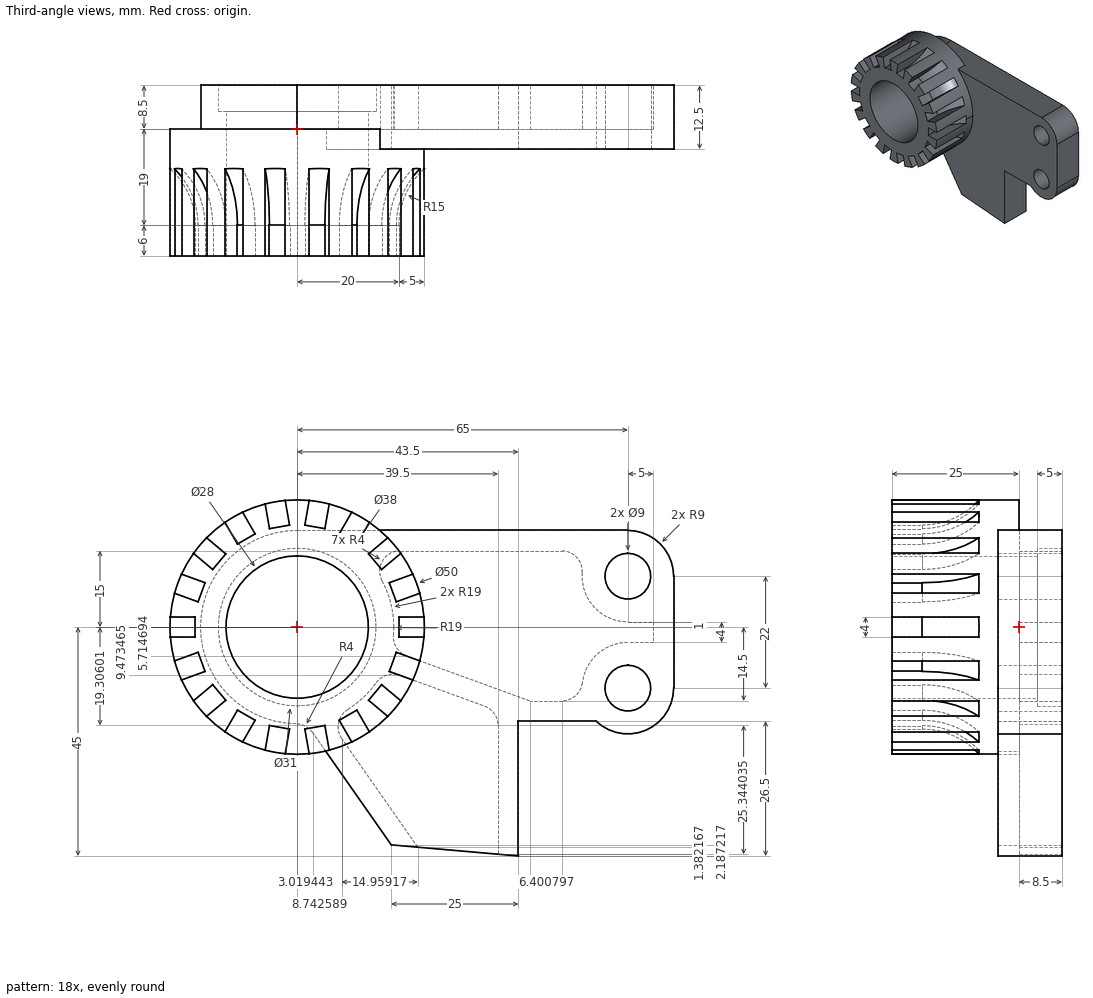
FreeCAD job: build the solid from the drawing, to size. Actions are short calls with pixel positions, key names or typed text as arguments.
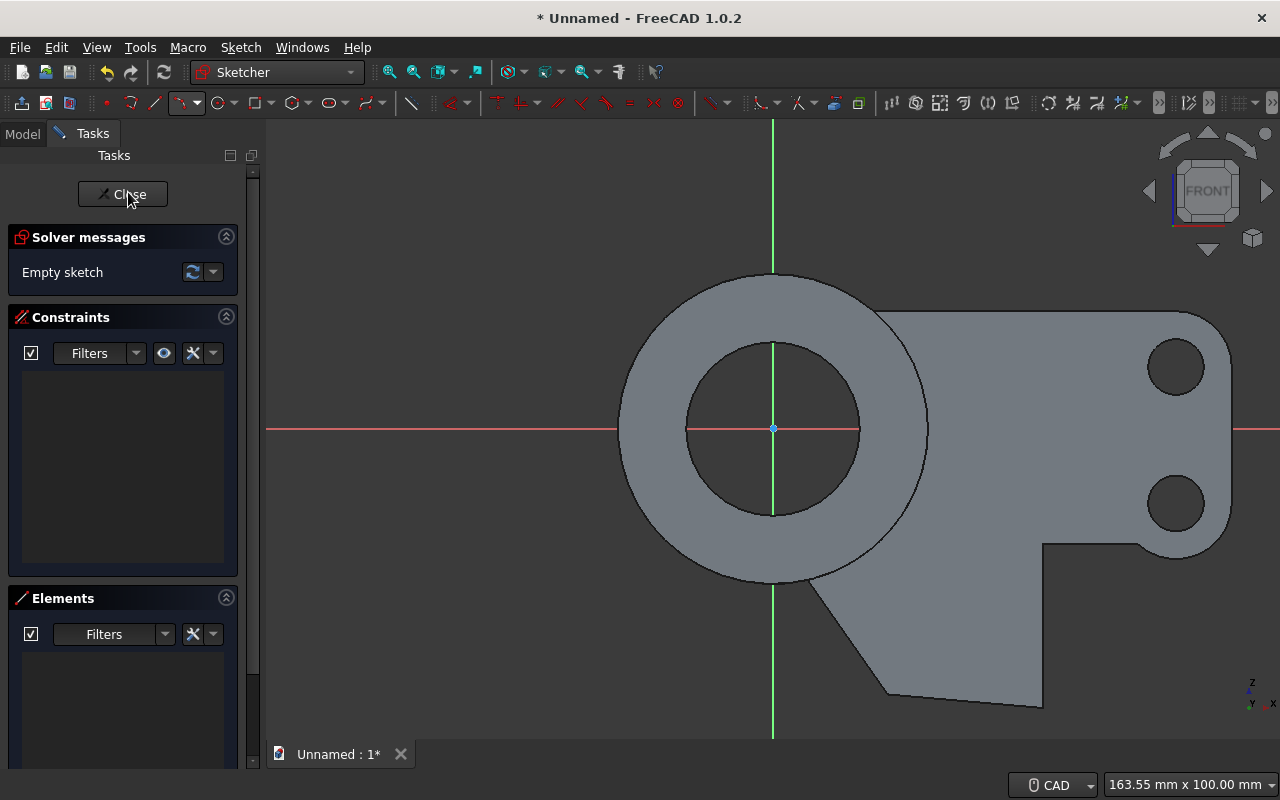
click(70, 104)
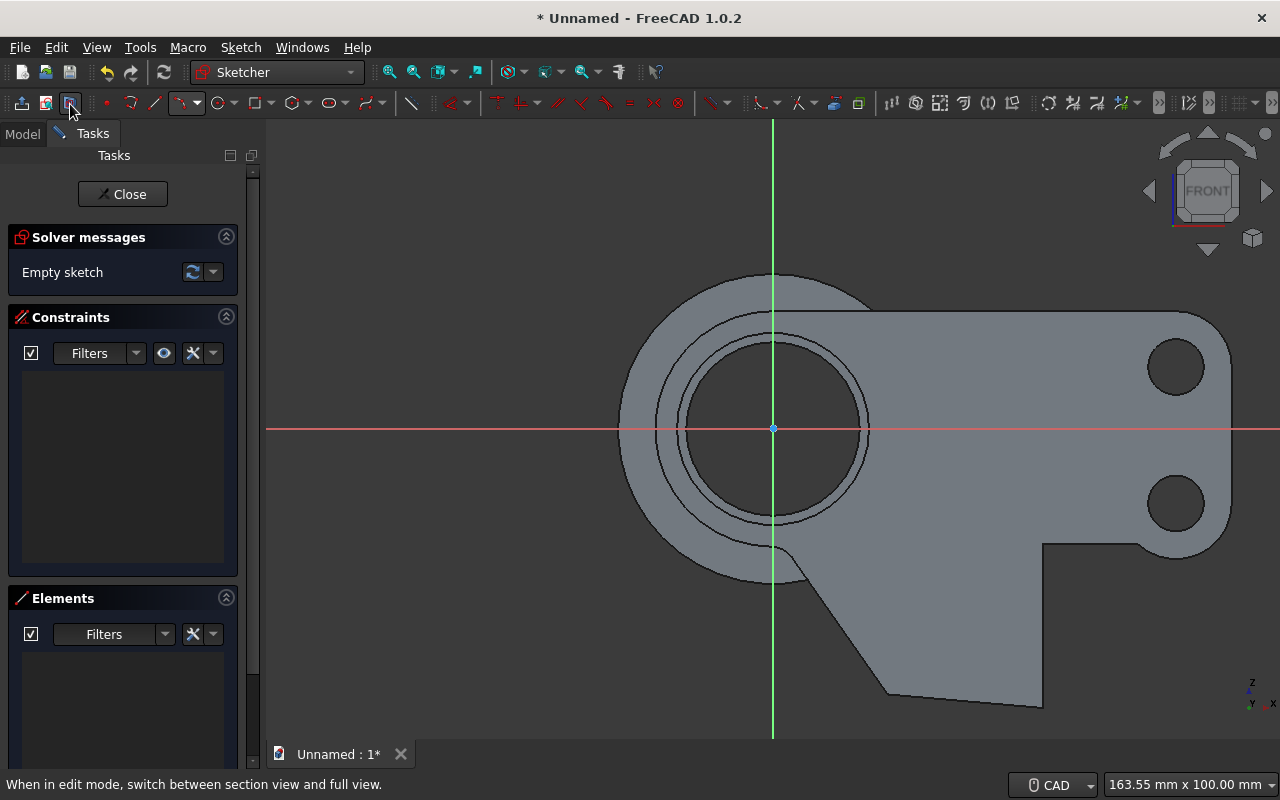
scroll(294, 147, down, 1)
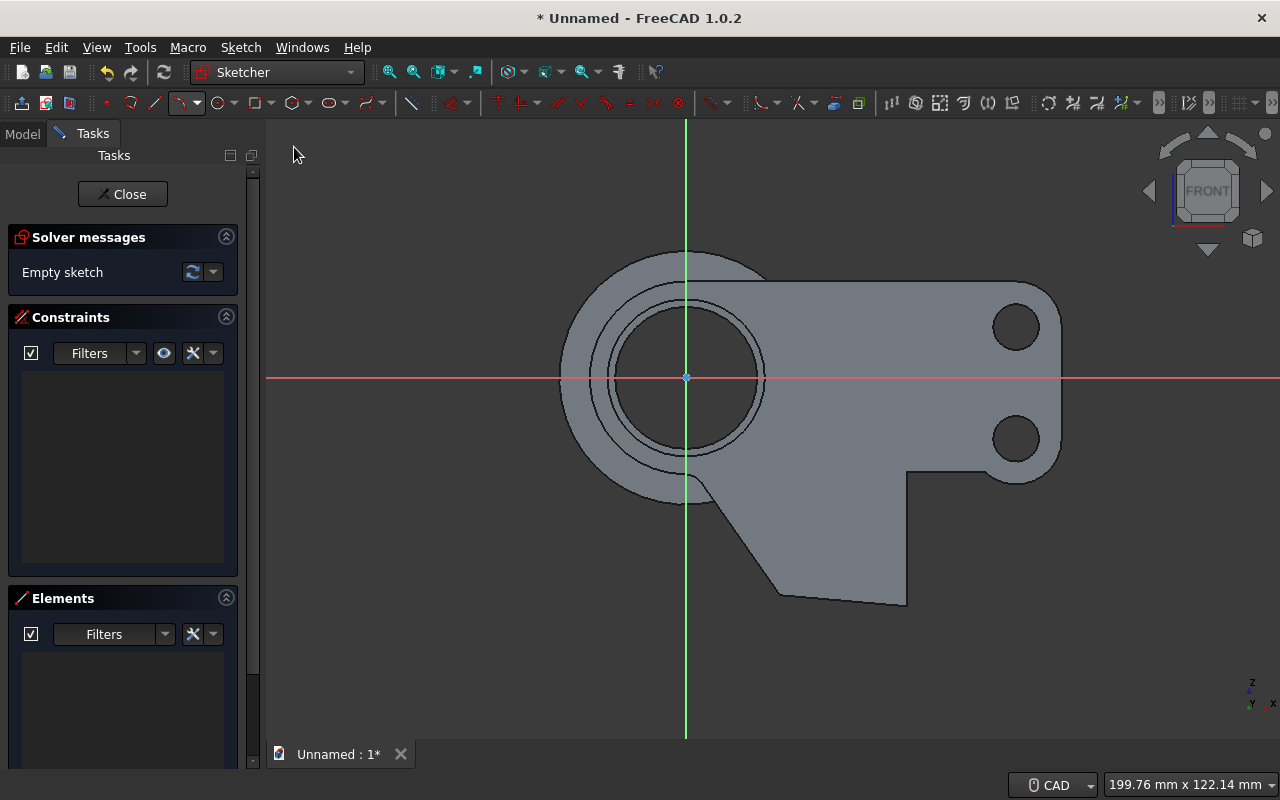
click(156, 104)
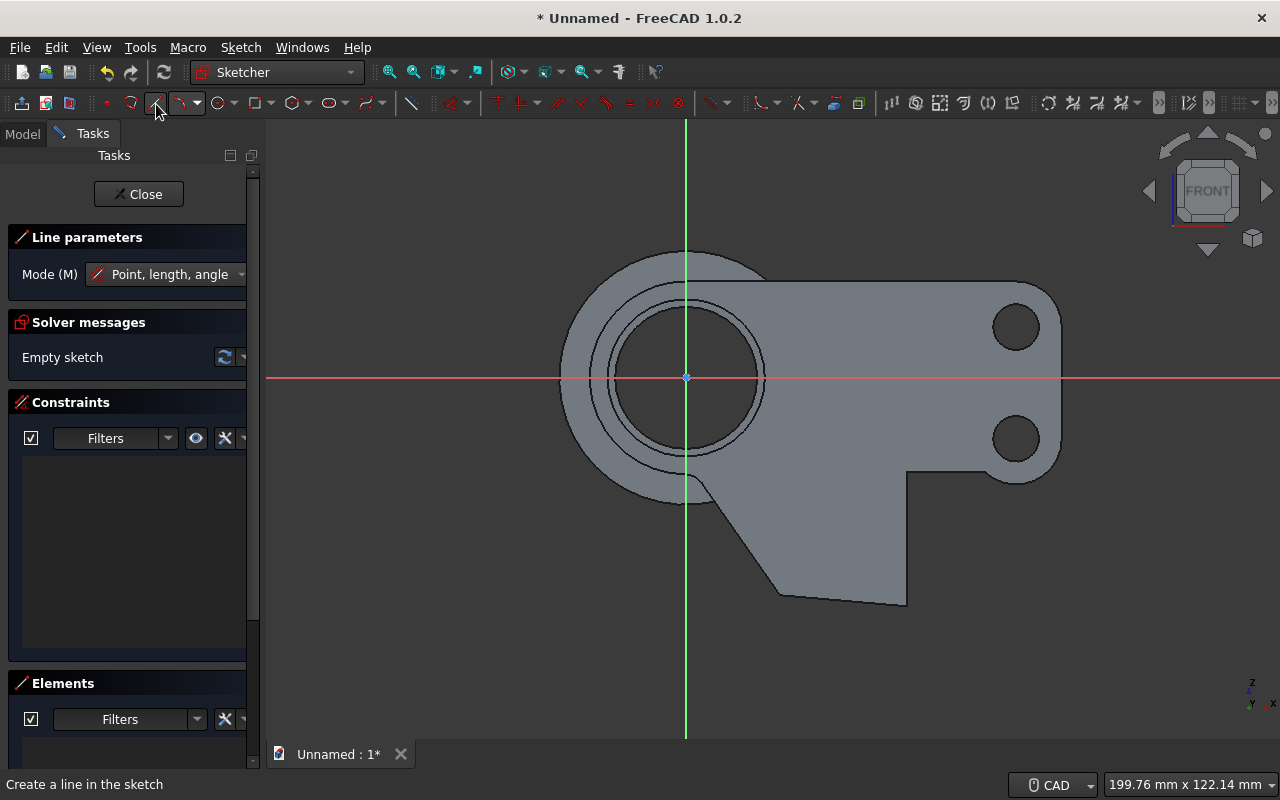
click(789, 302)
click(950, 302)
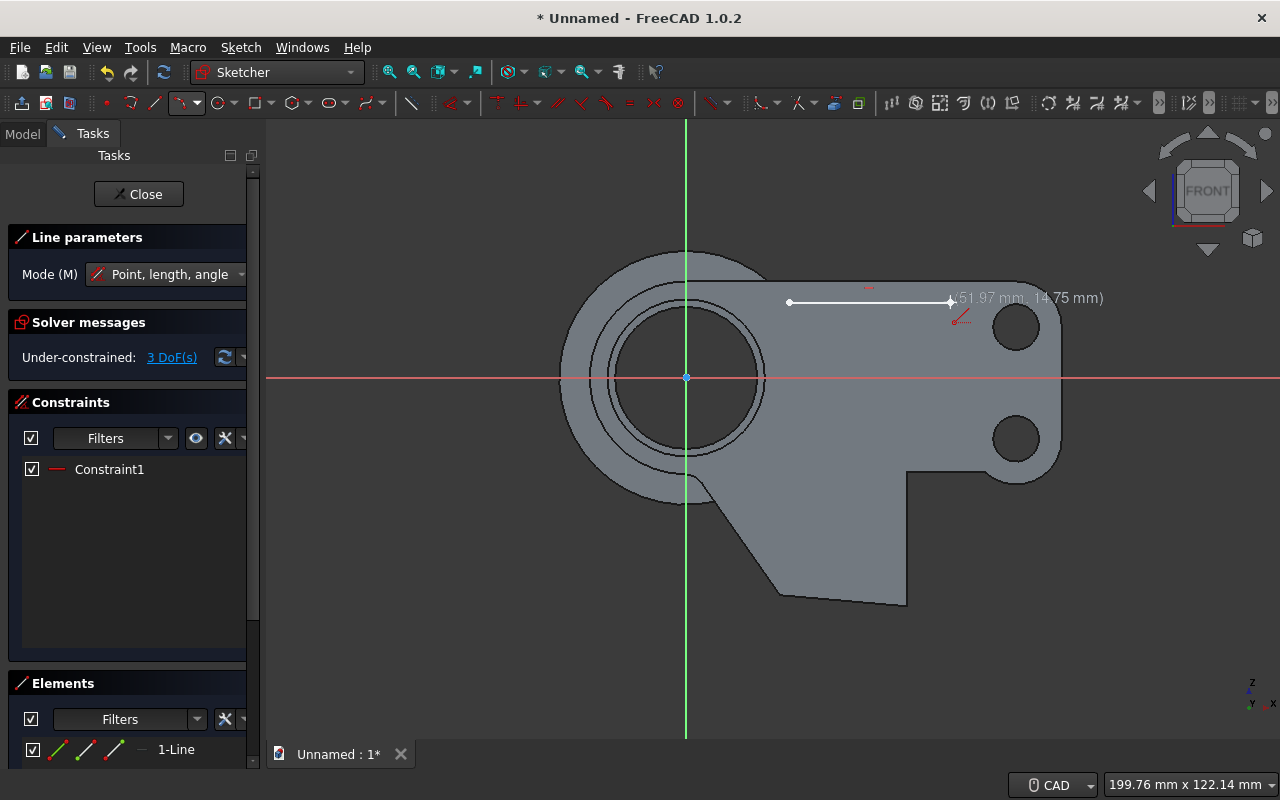
click(132, 104)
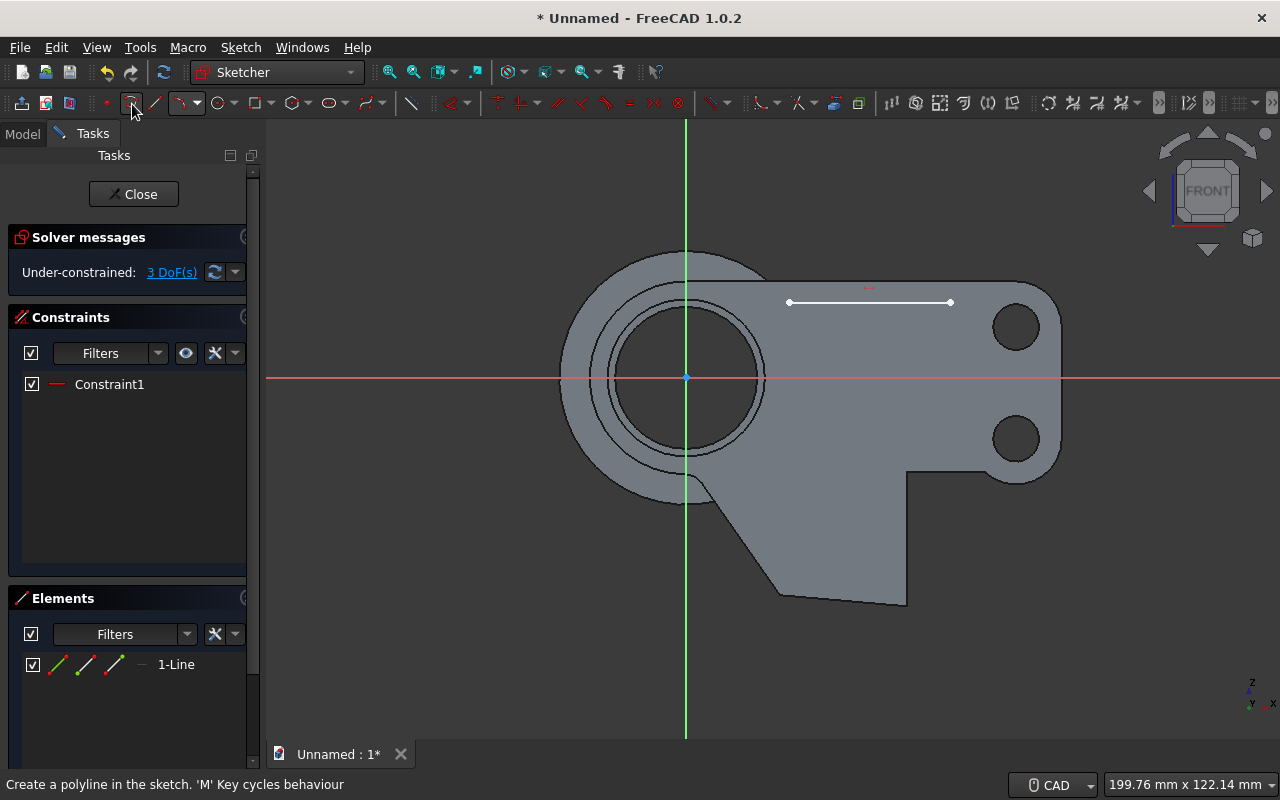
scroll(1016, 373, up, 6)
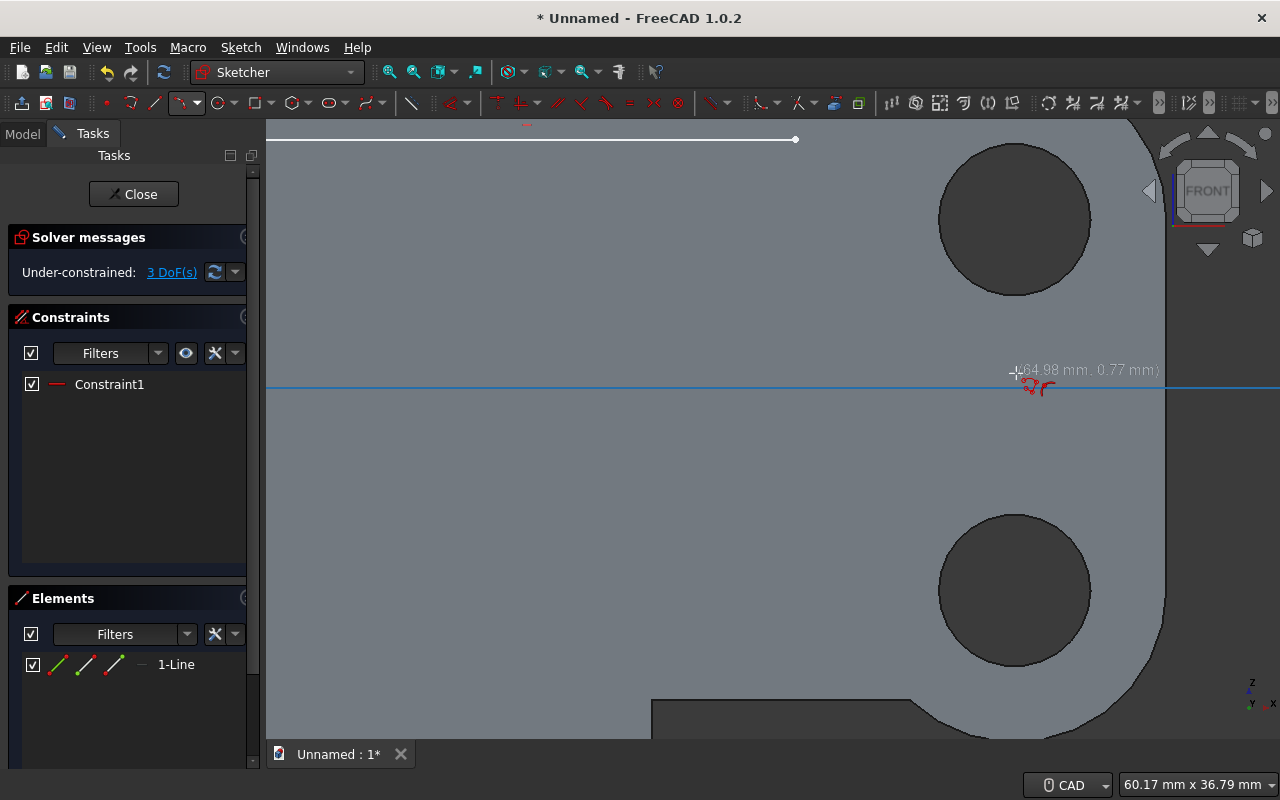
click(1015, 371)
click(1099, 371)
click(1099, 439)
click(1015, 439)
right_click(1015, 439)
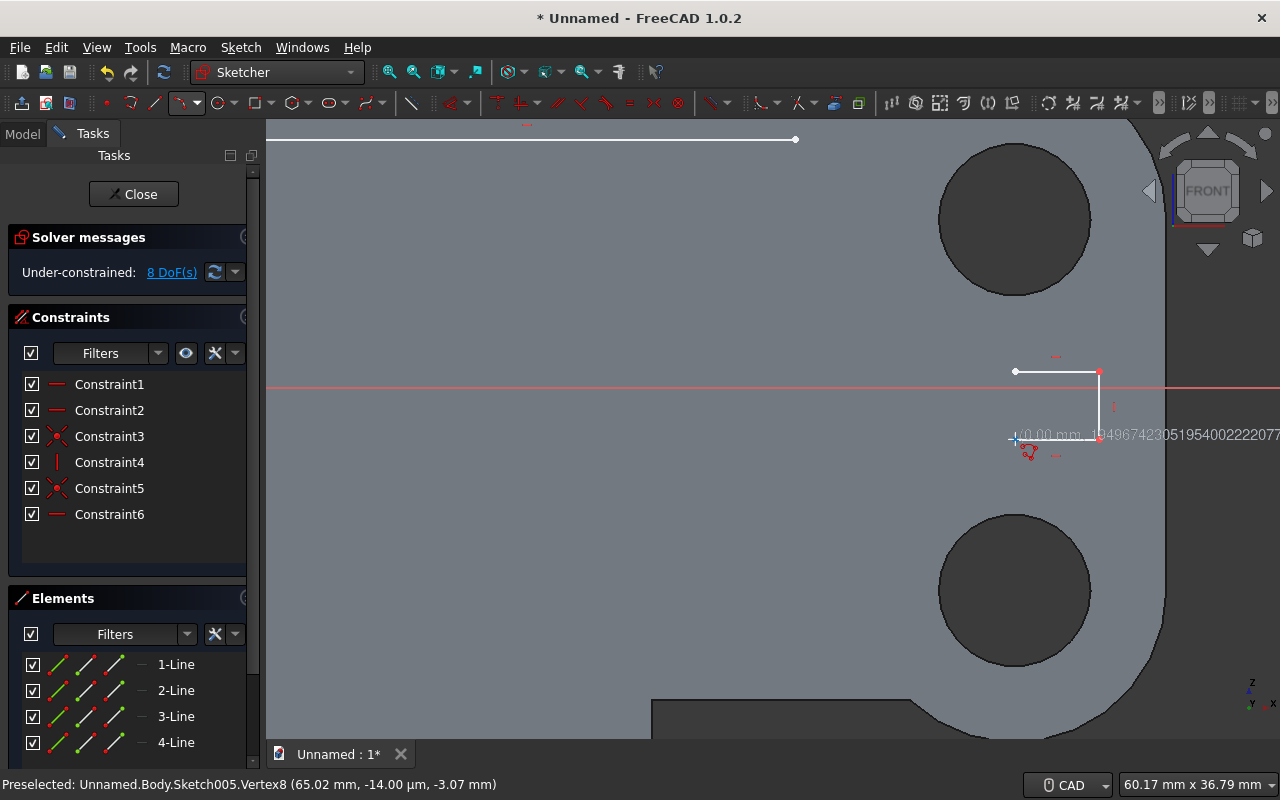
click(797, 633)
click(689, 633)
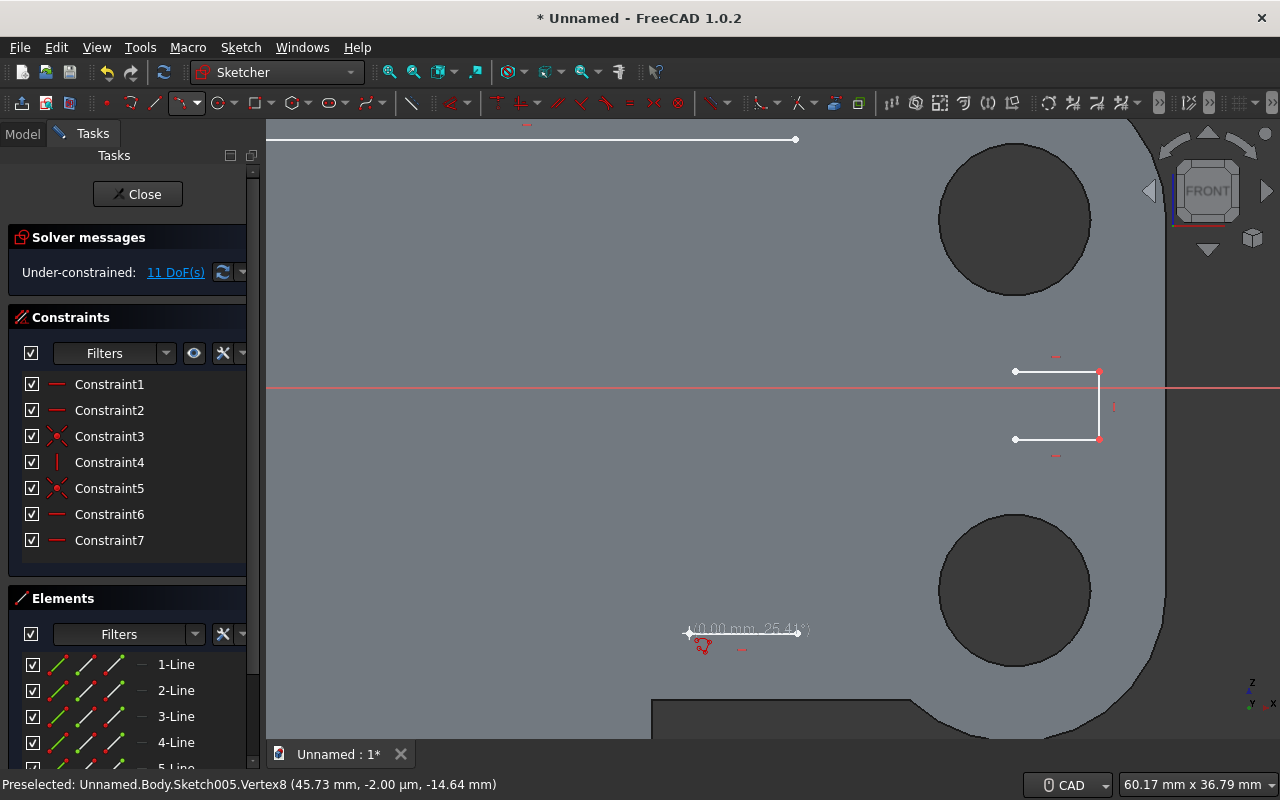
scroll(818, 307, down, 5)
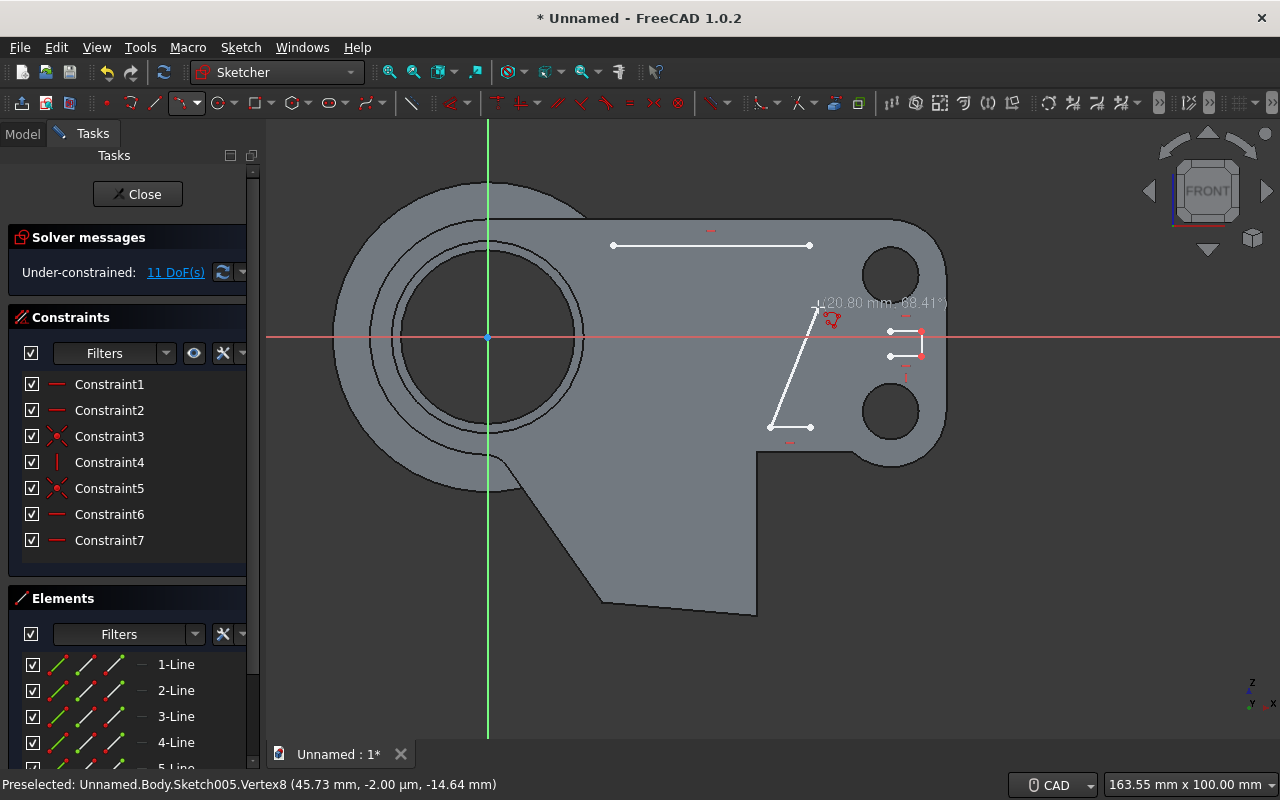
click(621, 373)
right_click(621, 373)